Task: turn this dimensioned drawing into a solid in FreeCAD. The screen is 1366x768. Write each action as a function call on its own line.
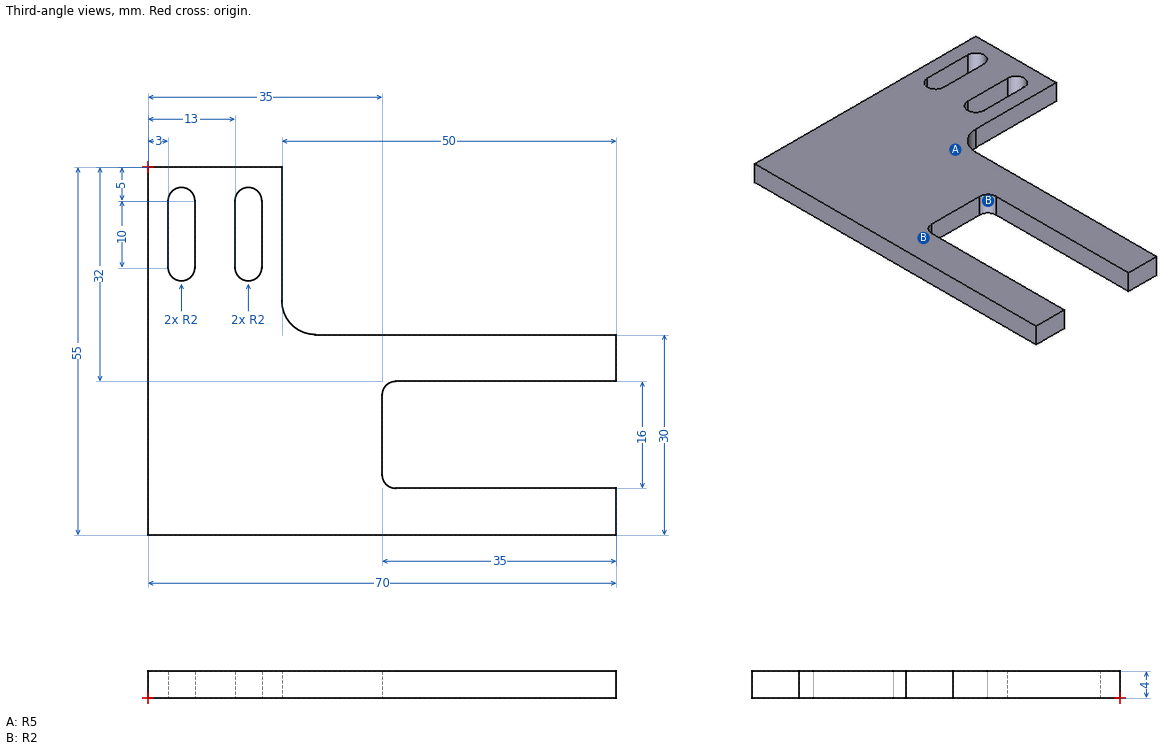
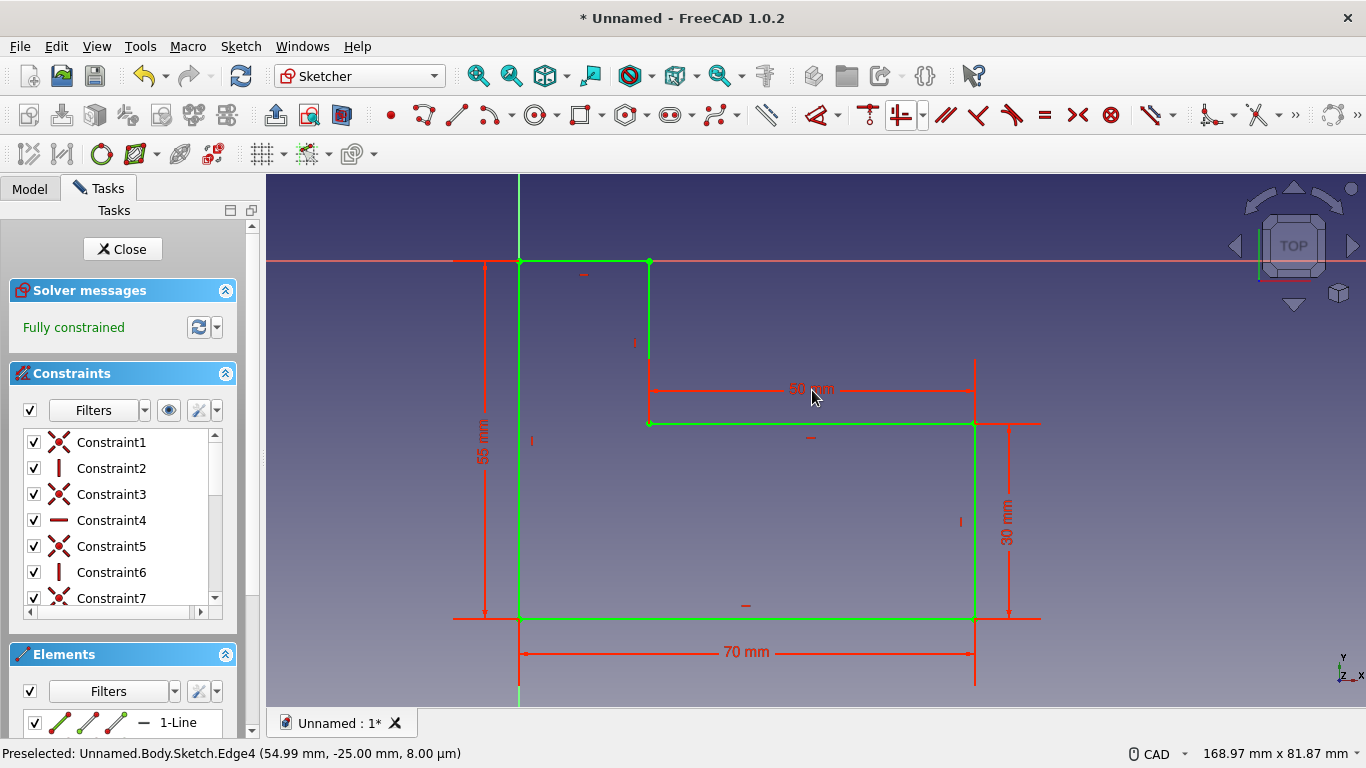
click(123, 249)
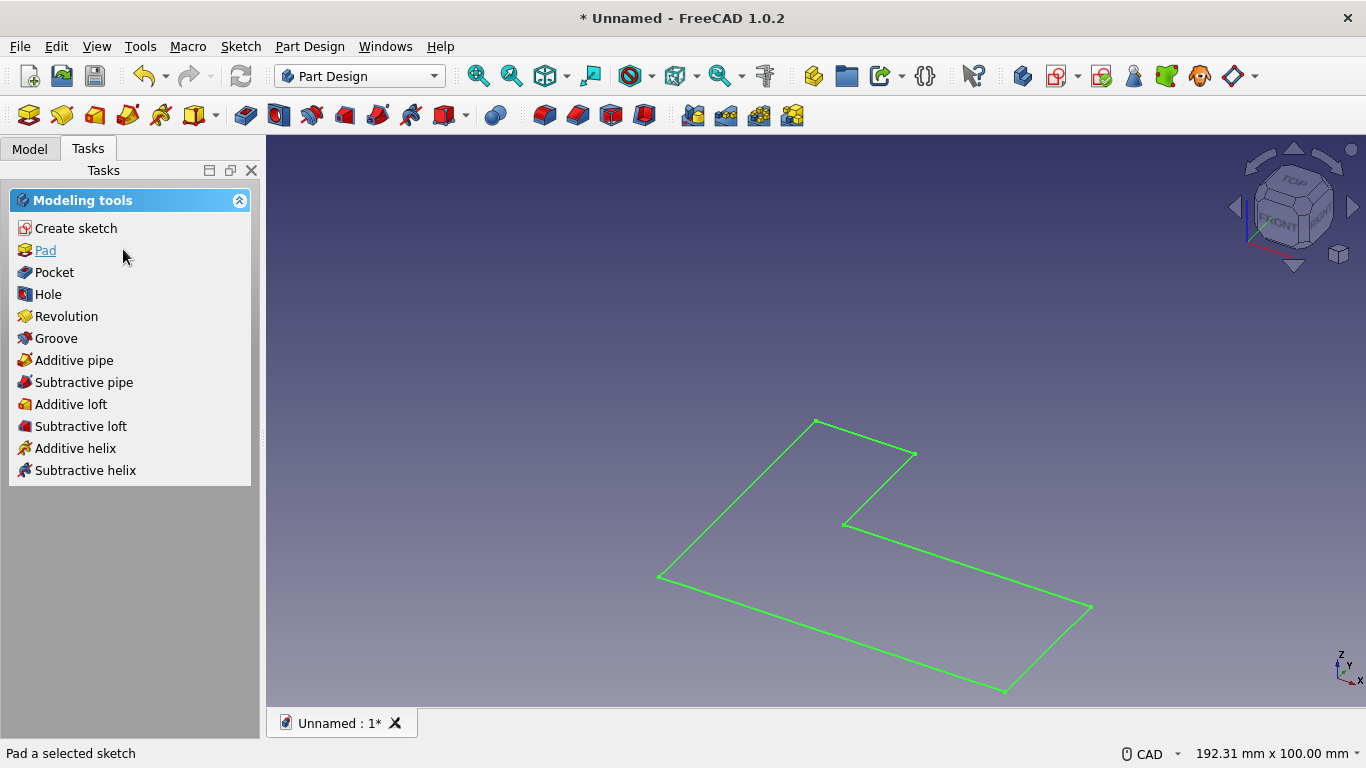
click(29, 116)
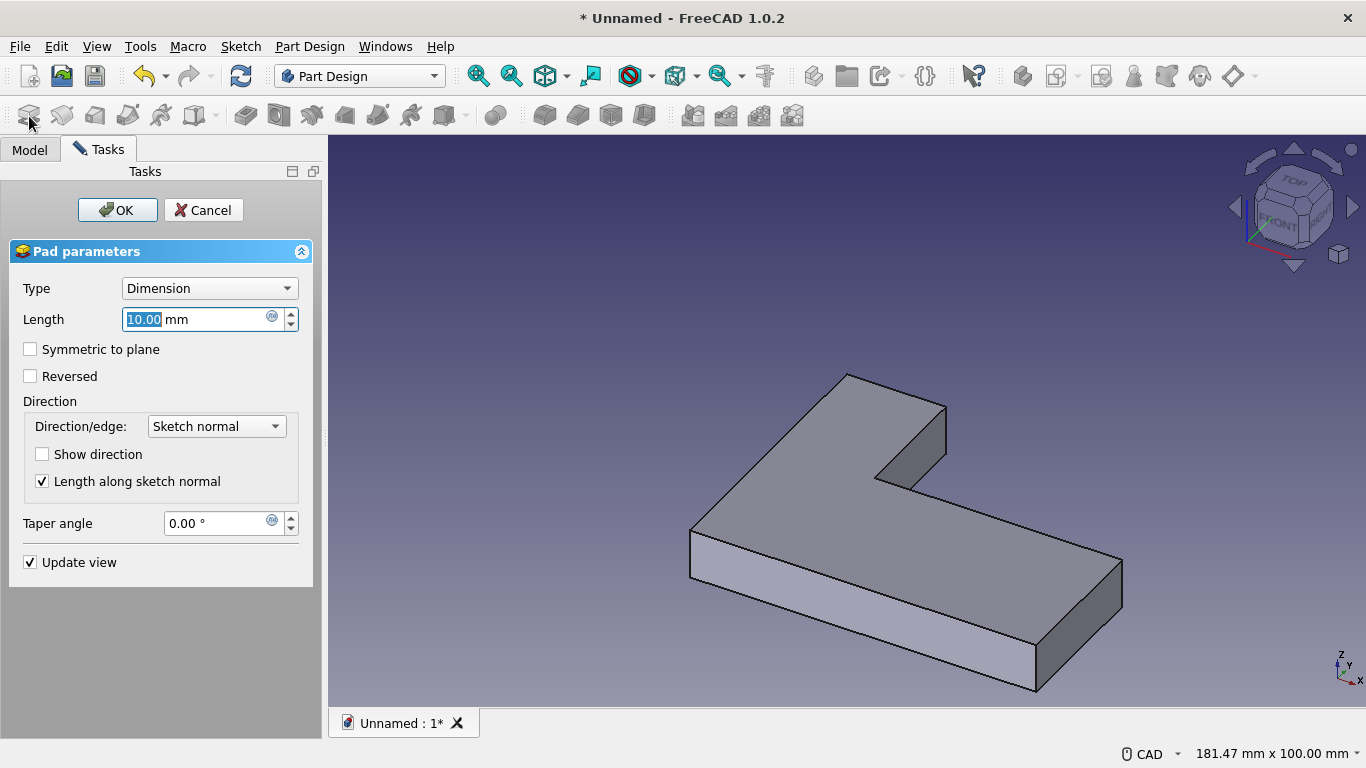
text(4)
key(Tab)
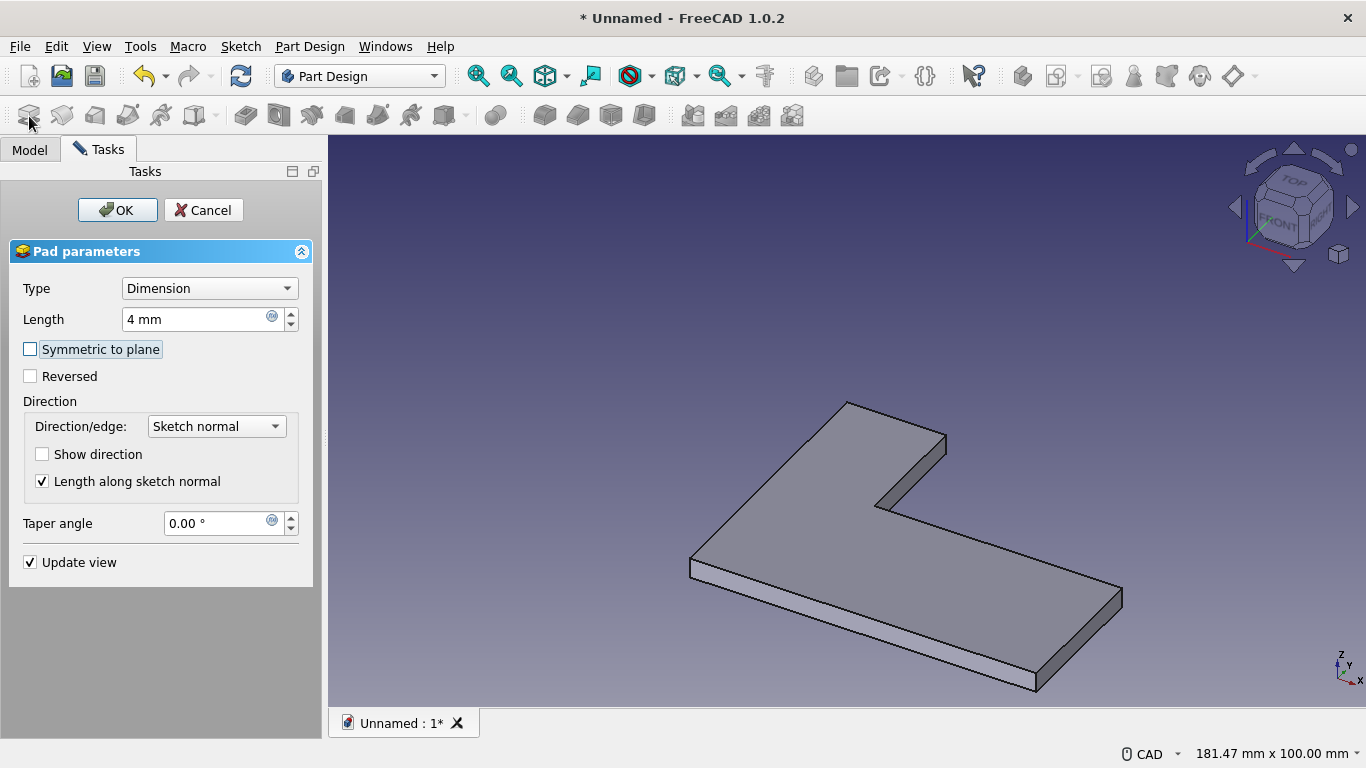
click(118, 210)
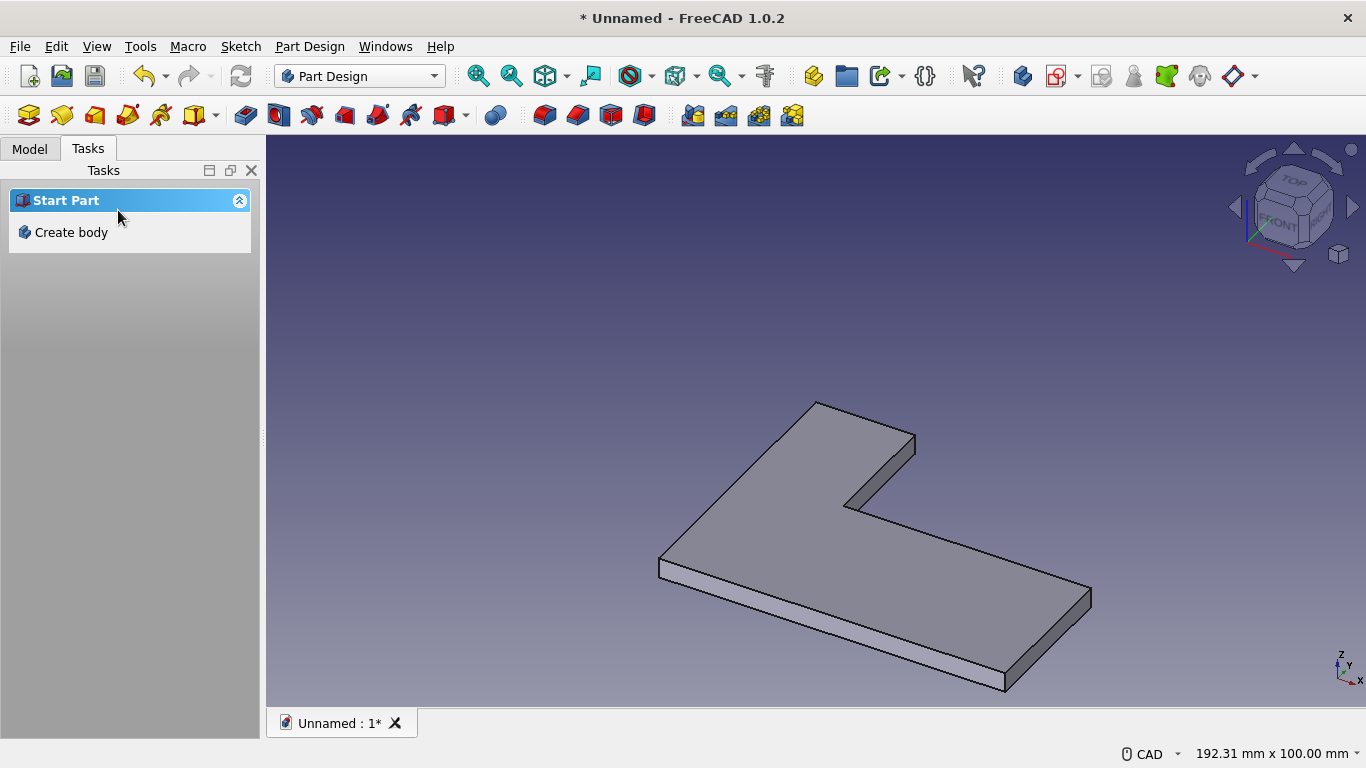
click(965, 614)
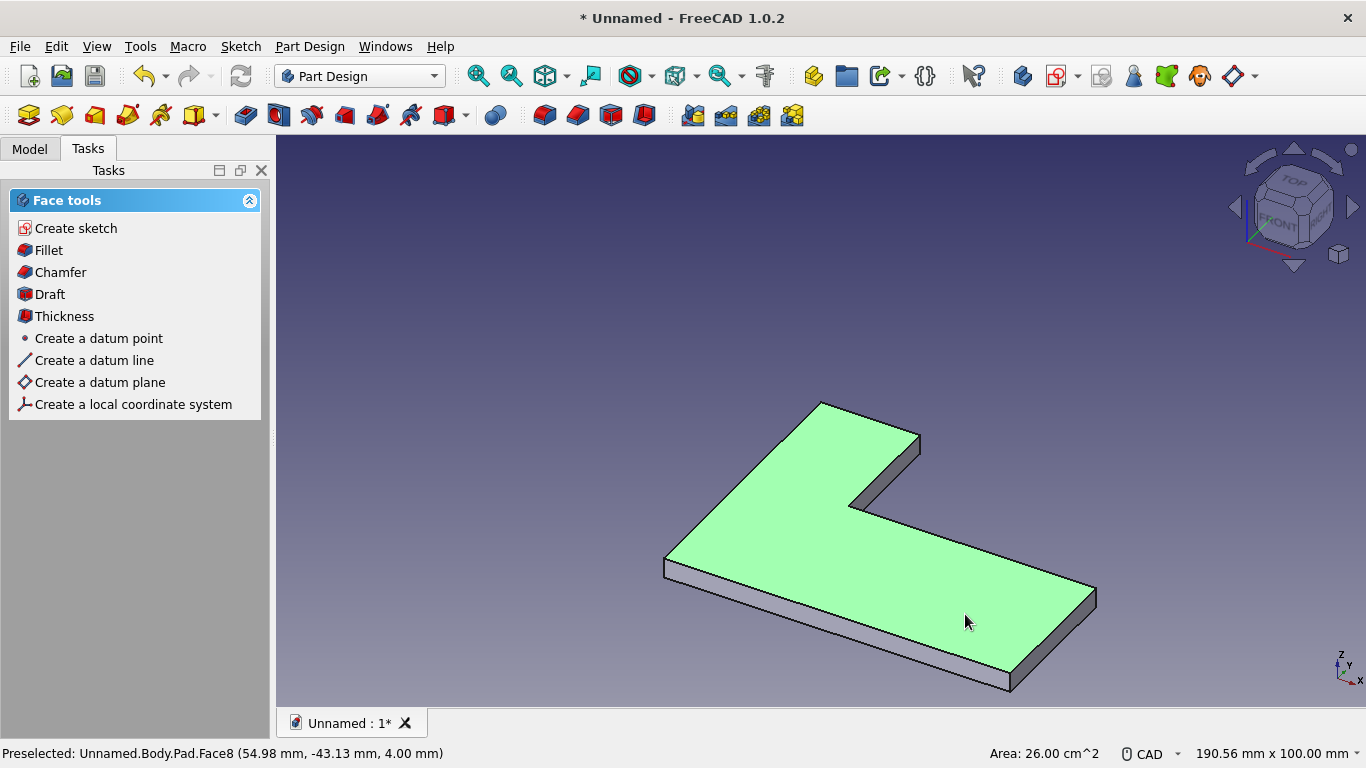
click(1056, 76)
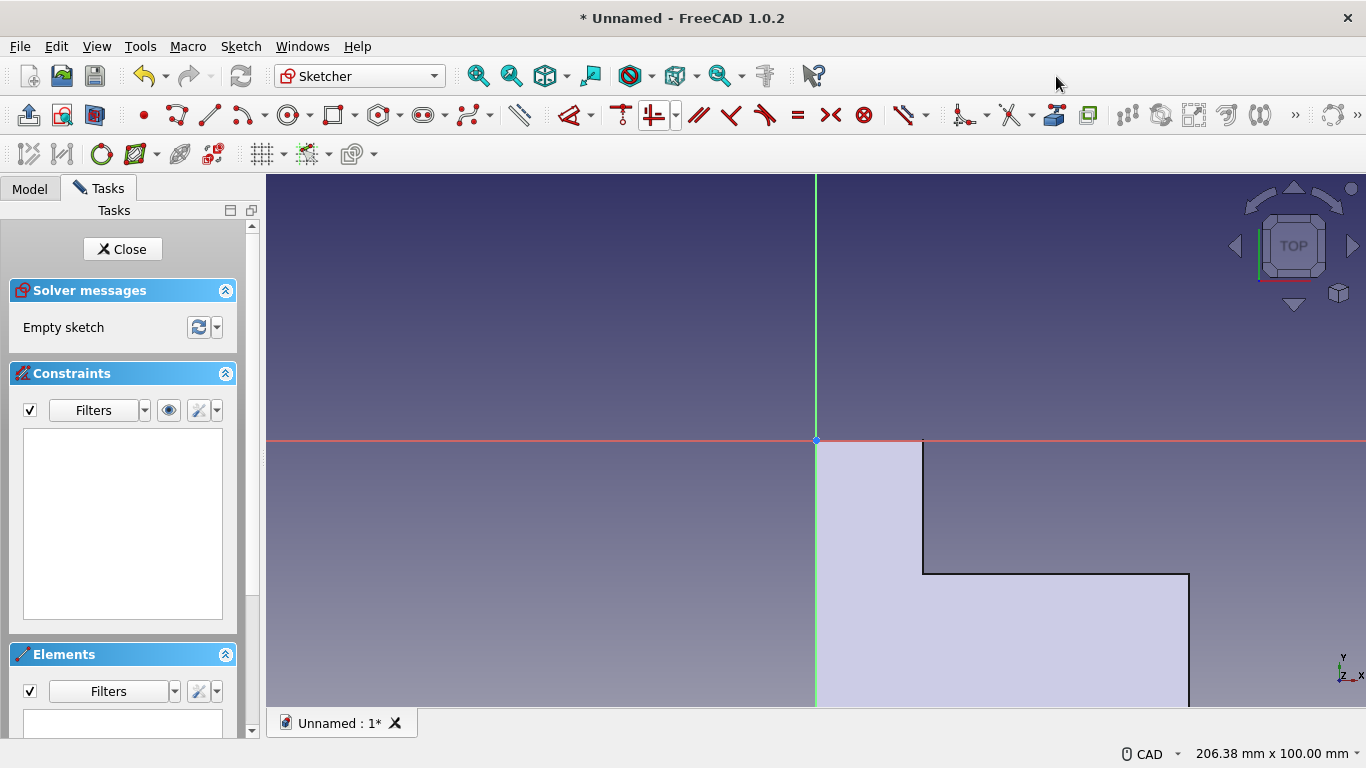
scroll(863, 501, up, 7)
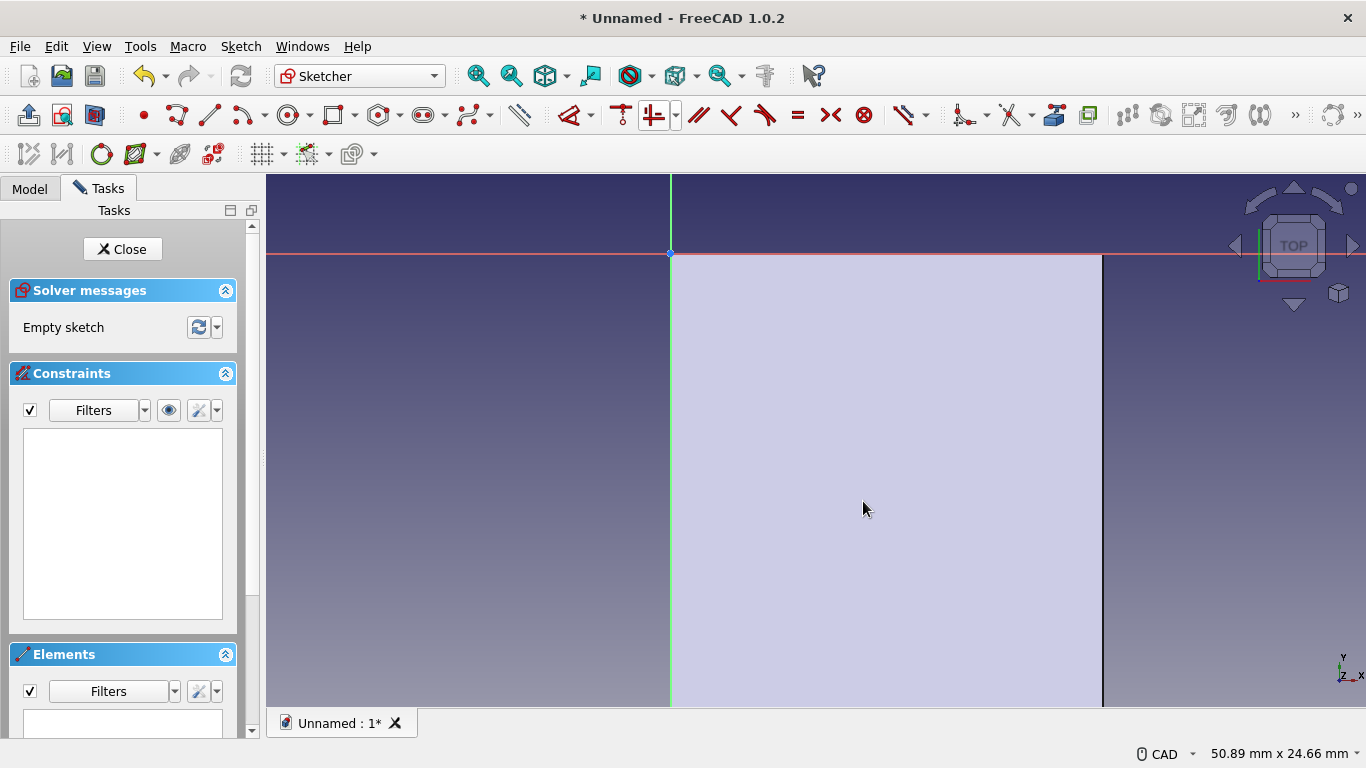
click(422, 116)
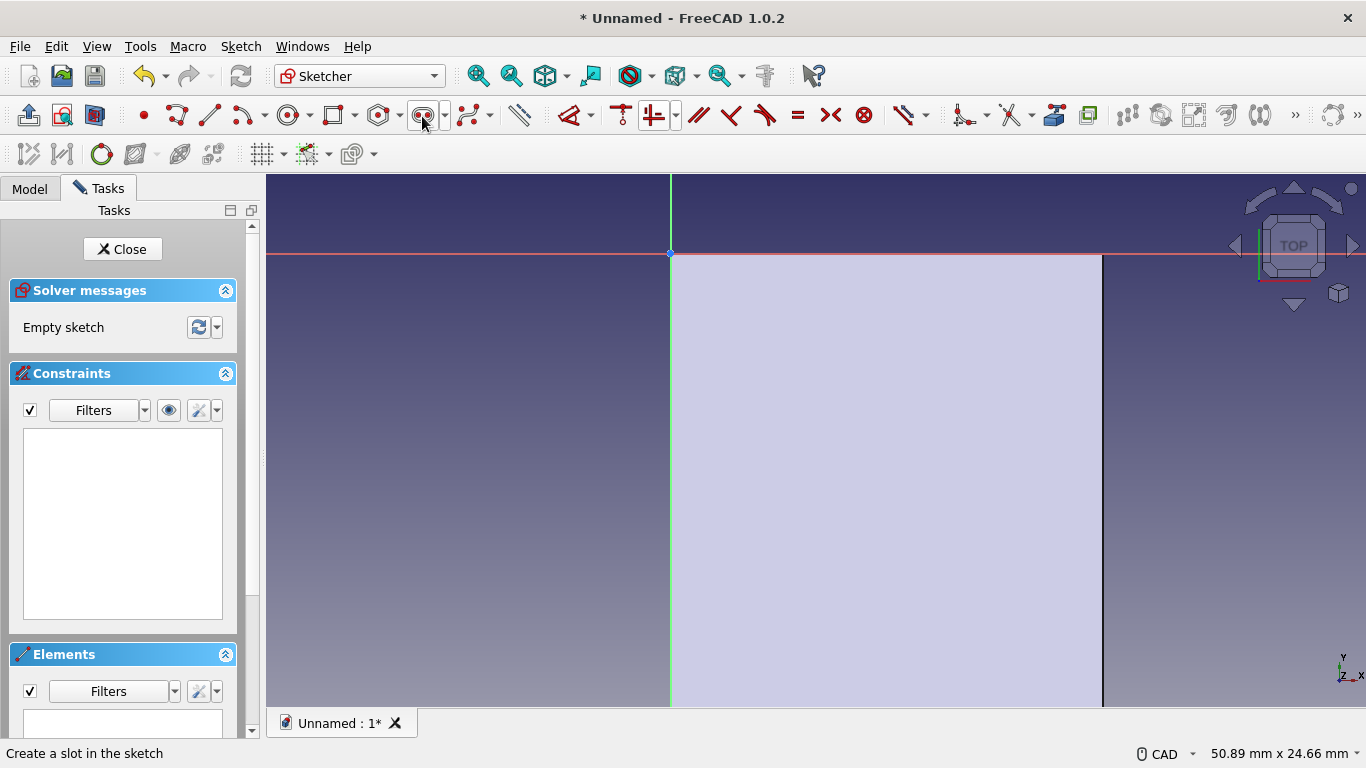
click(779, 578)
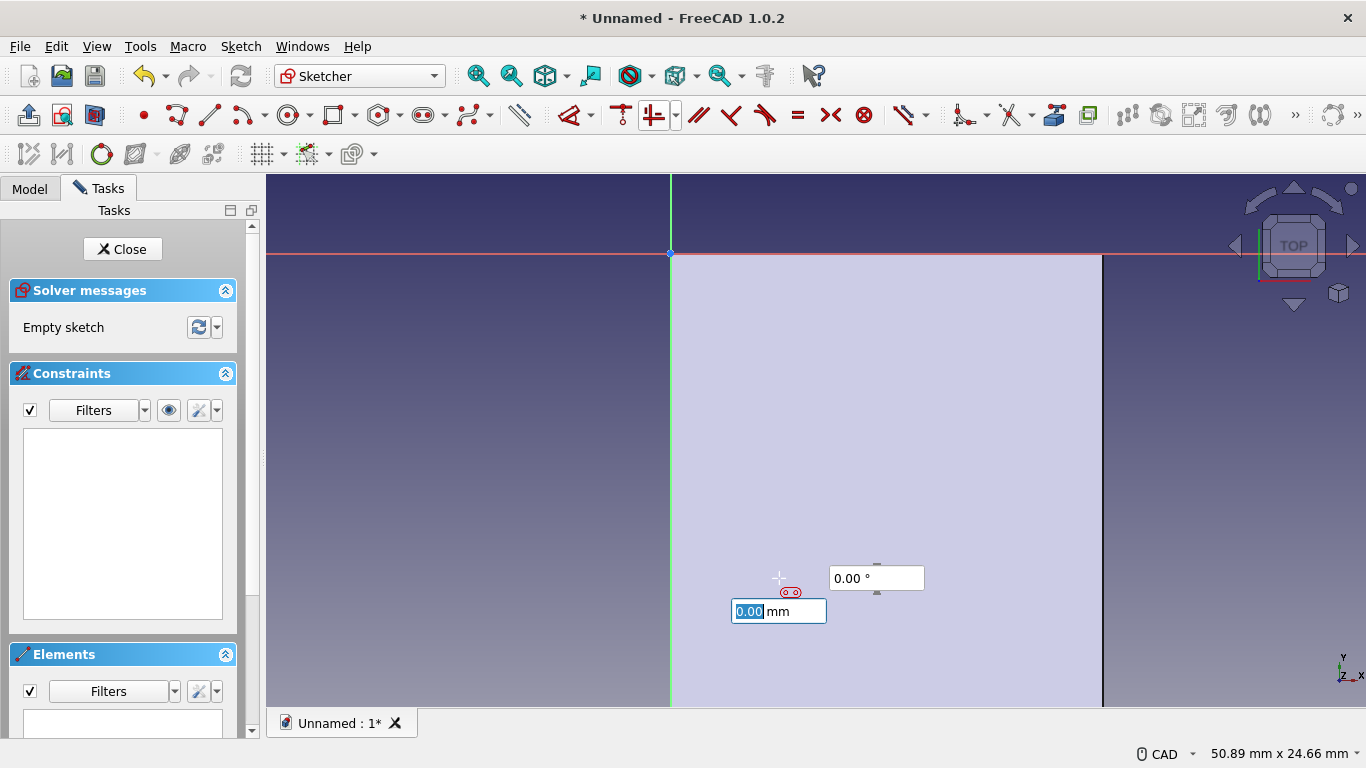
click(779, 362)